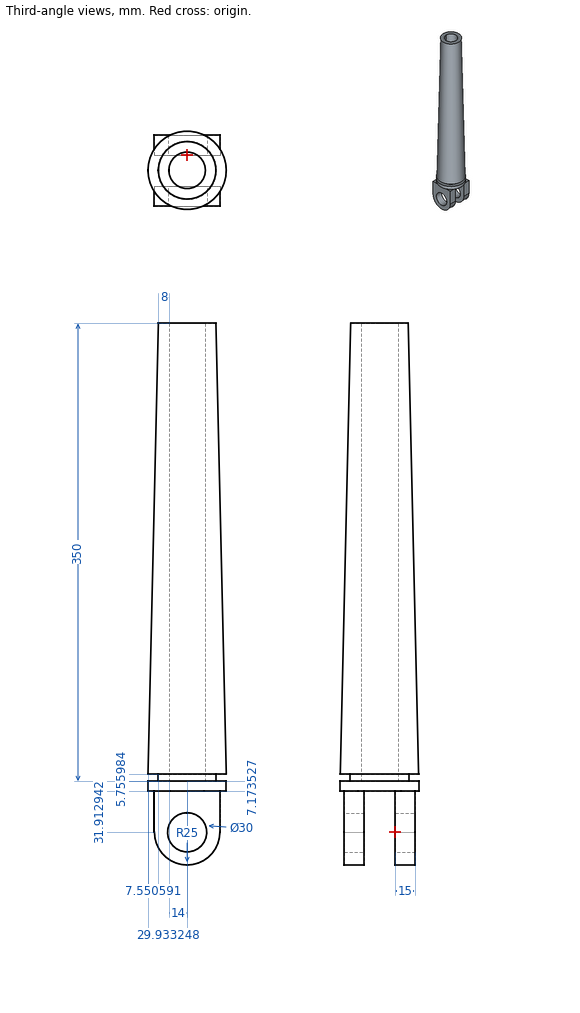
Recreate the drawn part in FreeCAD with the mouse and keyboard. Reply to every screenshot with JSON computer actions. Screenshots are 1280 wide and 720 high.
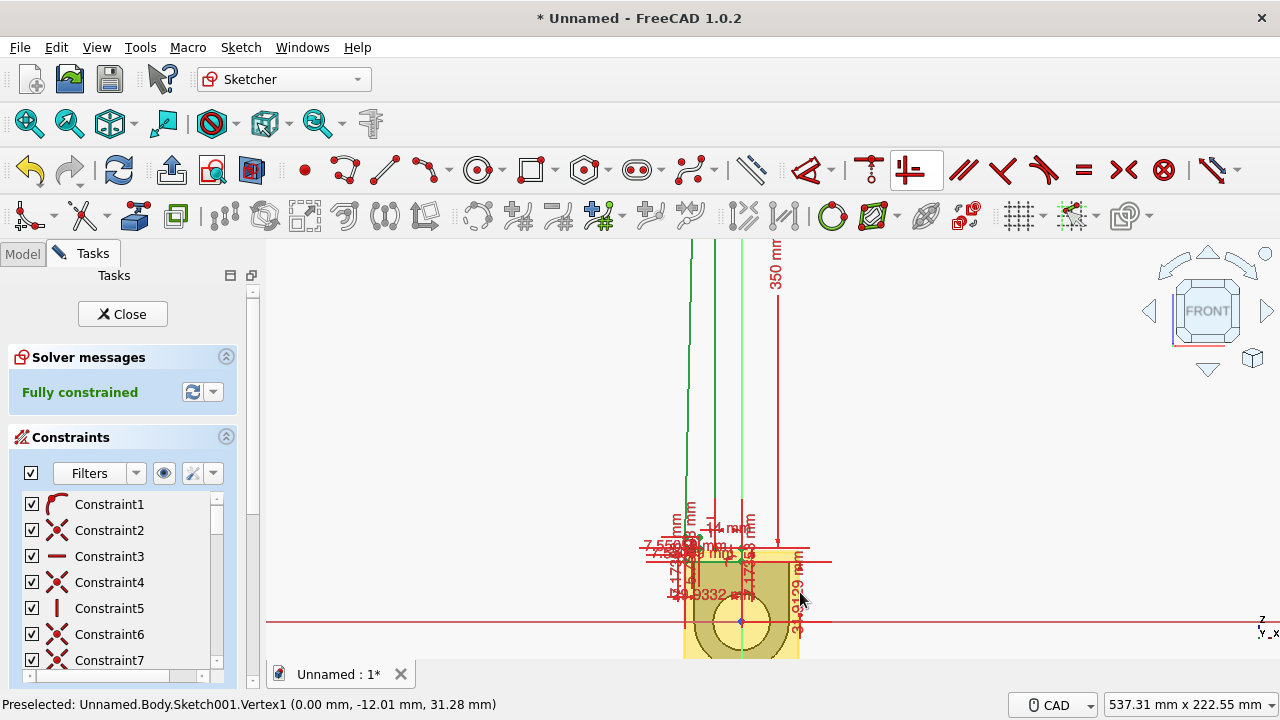
{"action": "left_click", "coordinate": [123, 314]}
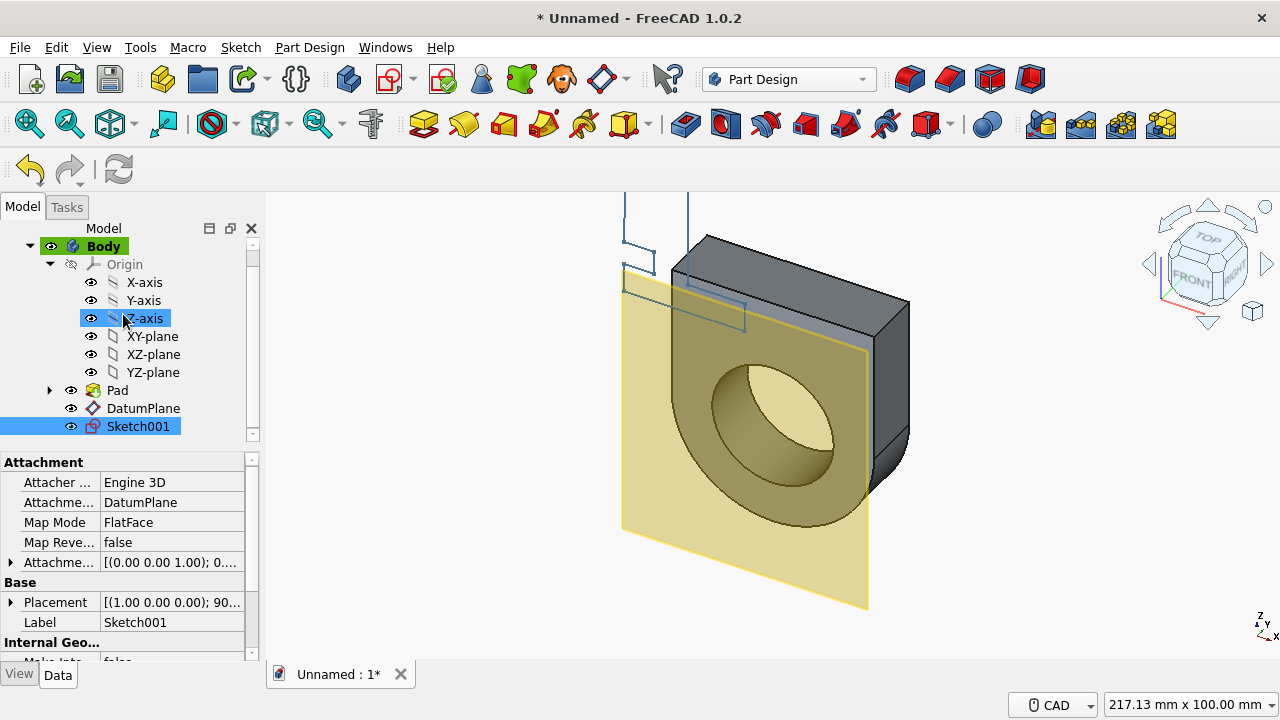
{"action": "left_click", "coordinate": [464, 124]}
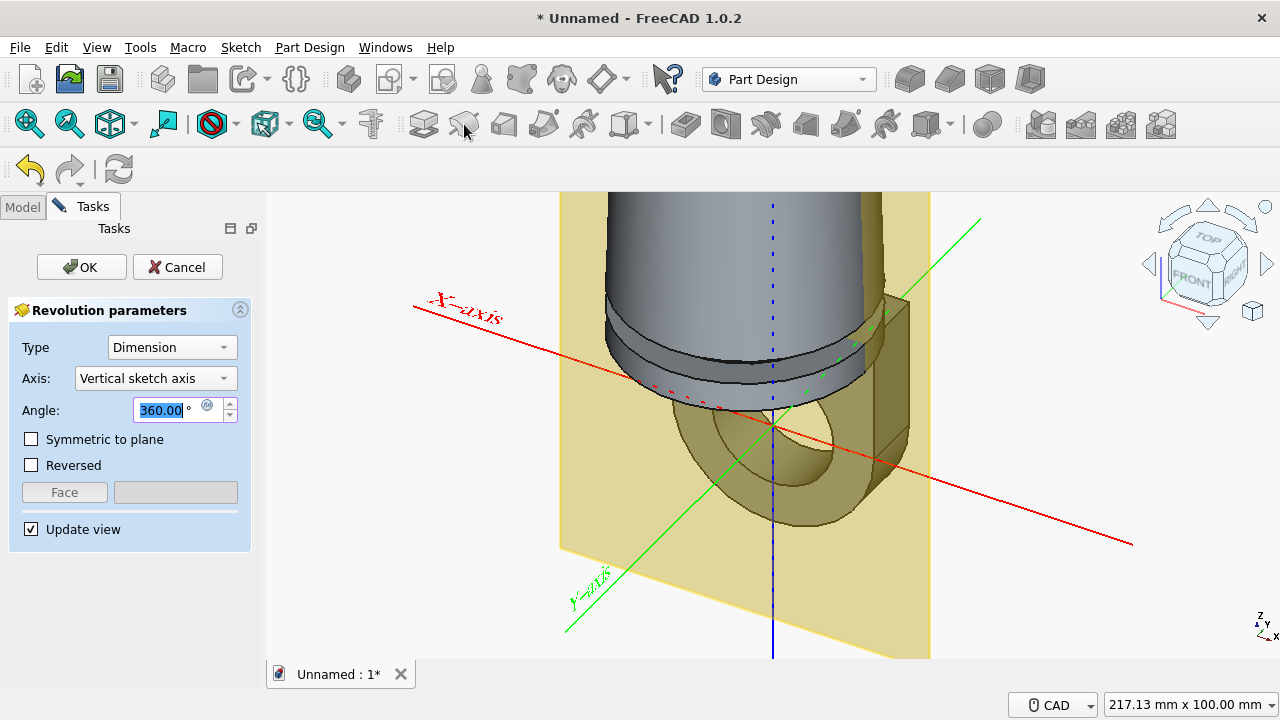
{"action": "left_click", "coordinate": [82, 267]}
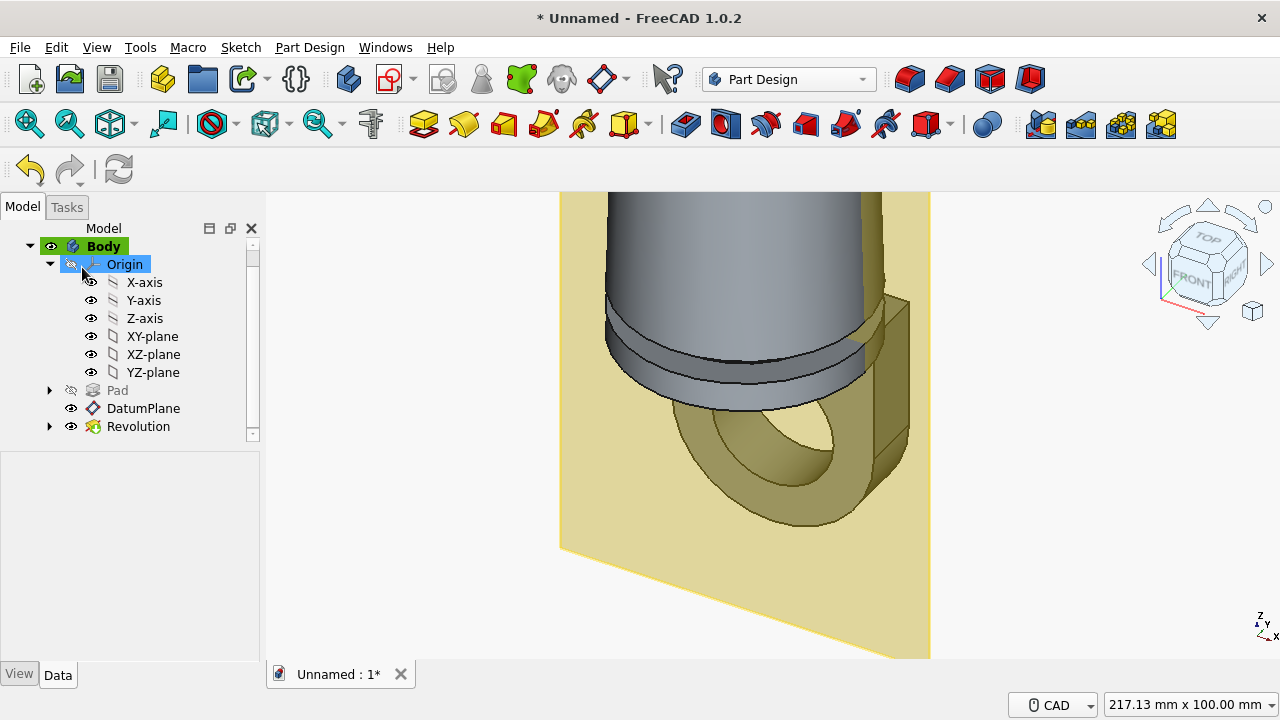
{"action": "left_click", "coordinate": [116, 408]}
{"action": "key", "text": "space"}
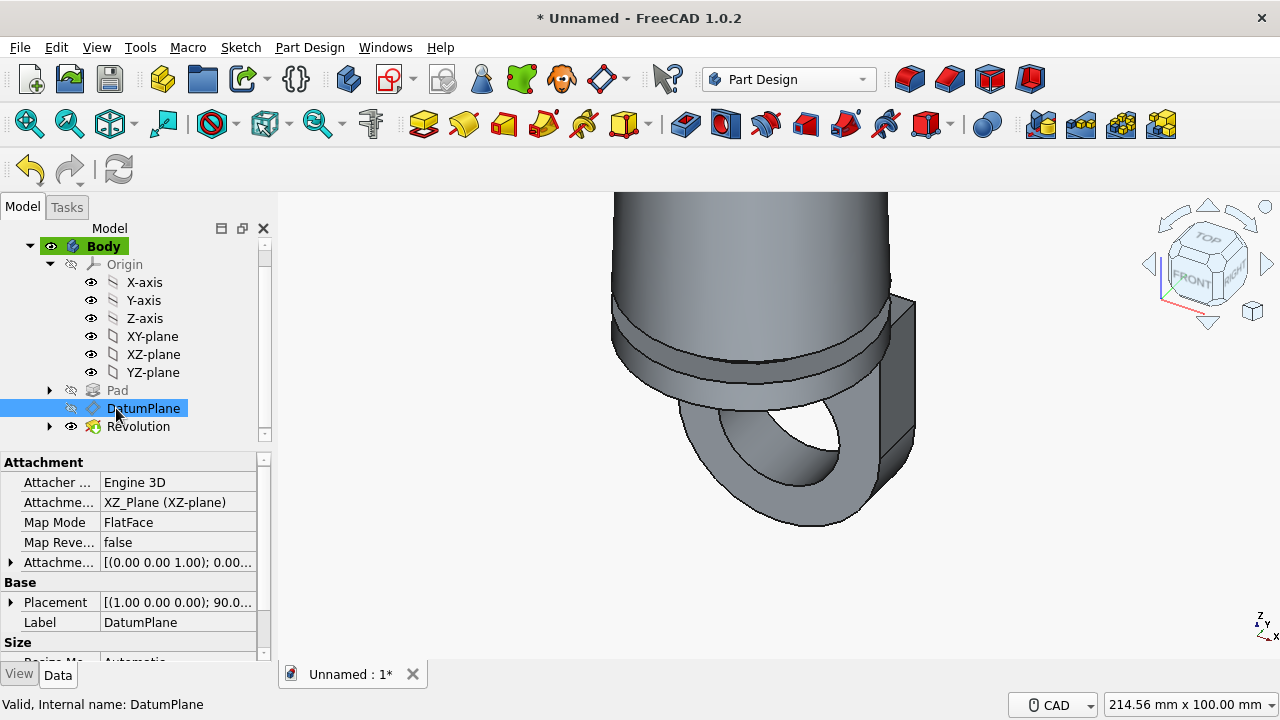
{"action": "left_click", "coordinate": [30, 124]}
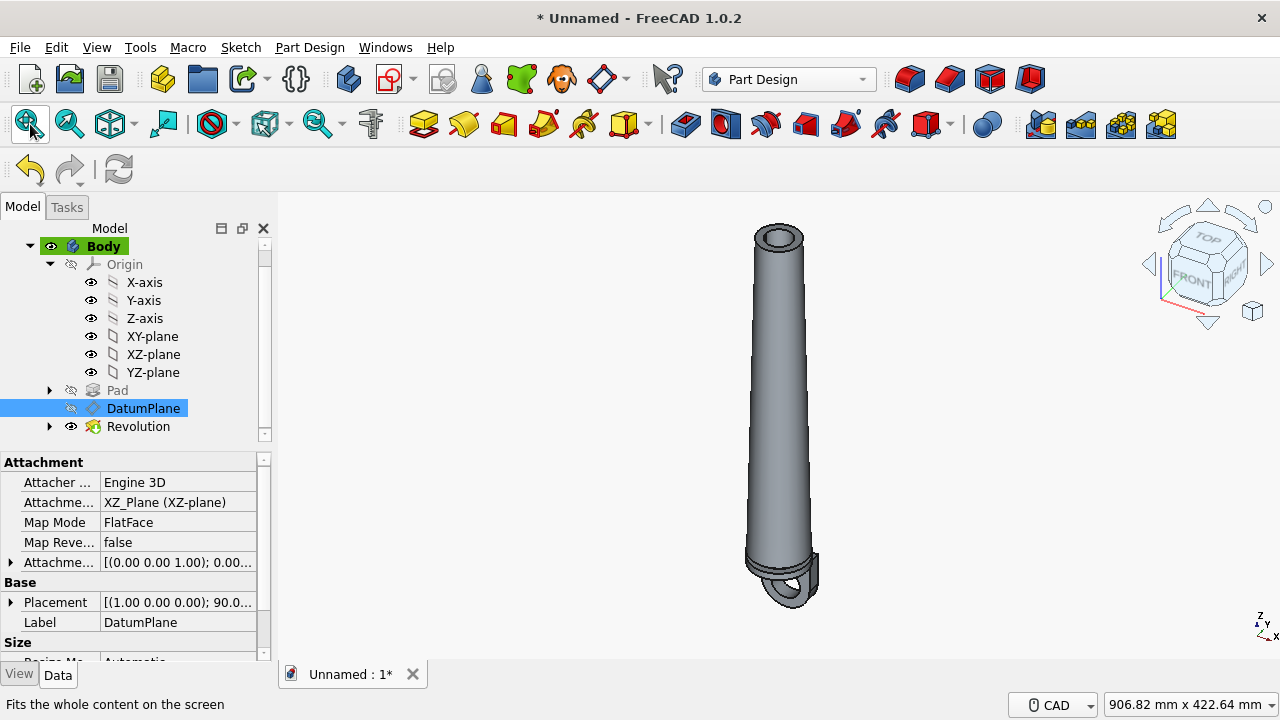
{"action": "left_click", "coordinate": [136, 354]}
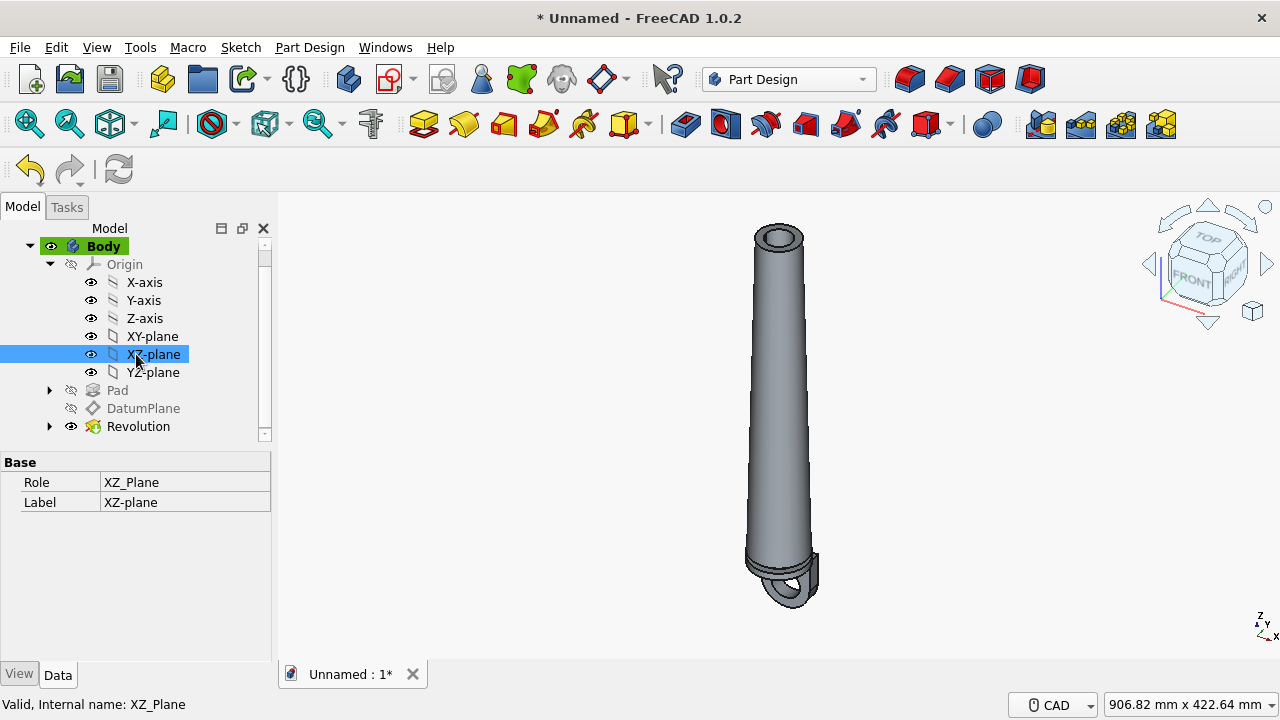
{"action": "left_click", "coordinate": [602, 80]}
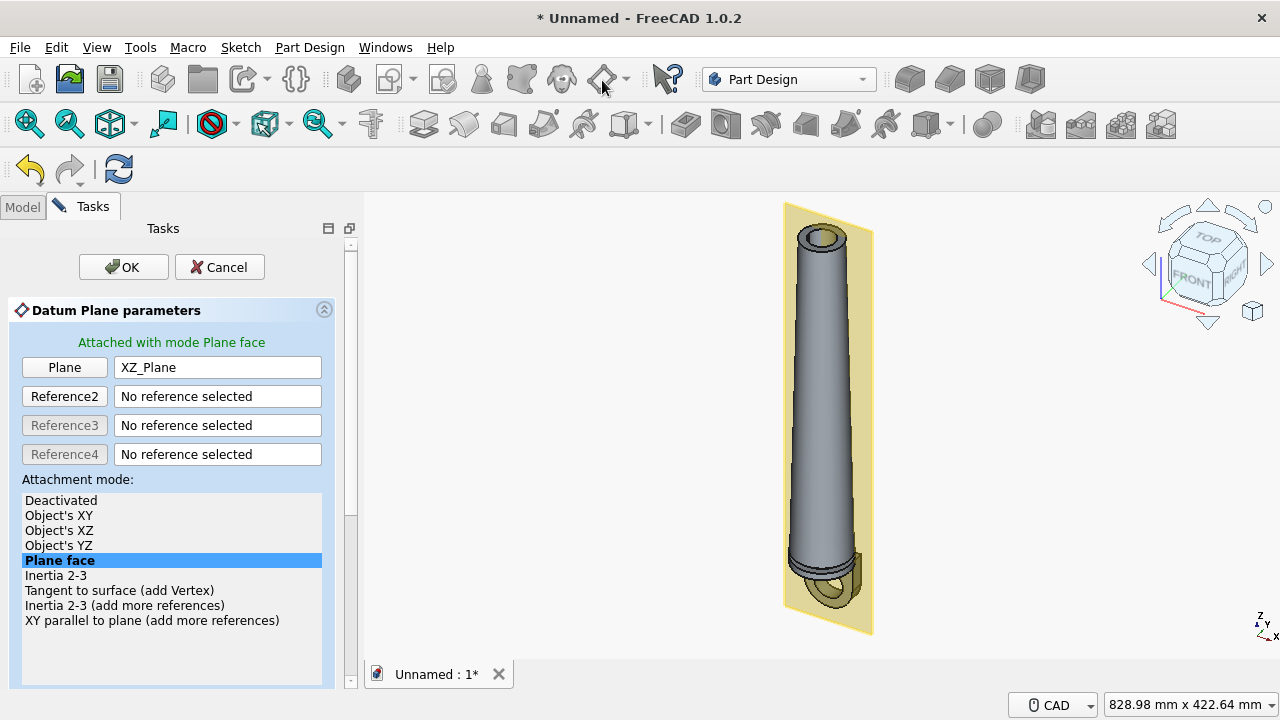
{"action": "scroll", "coordinate": [351, 463], "scroll_direction": "down", "scroll_amount": 3}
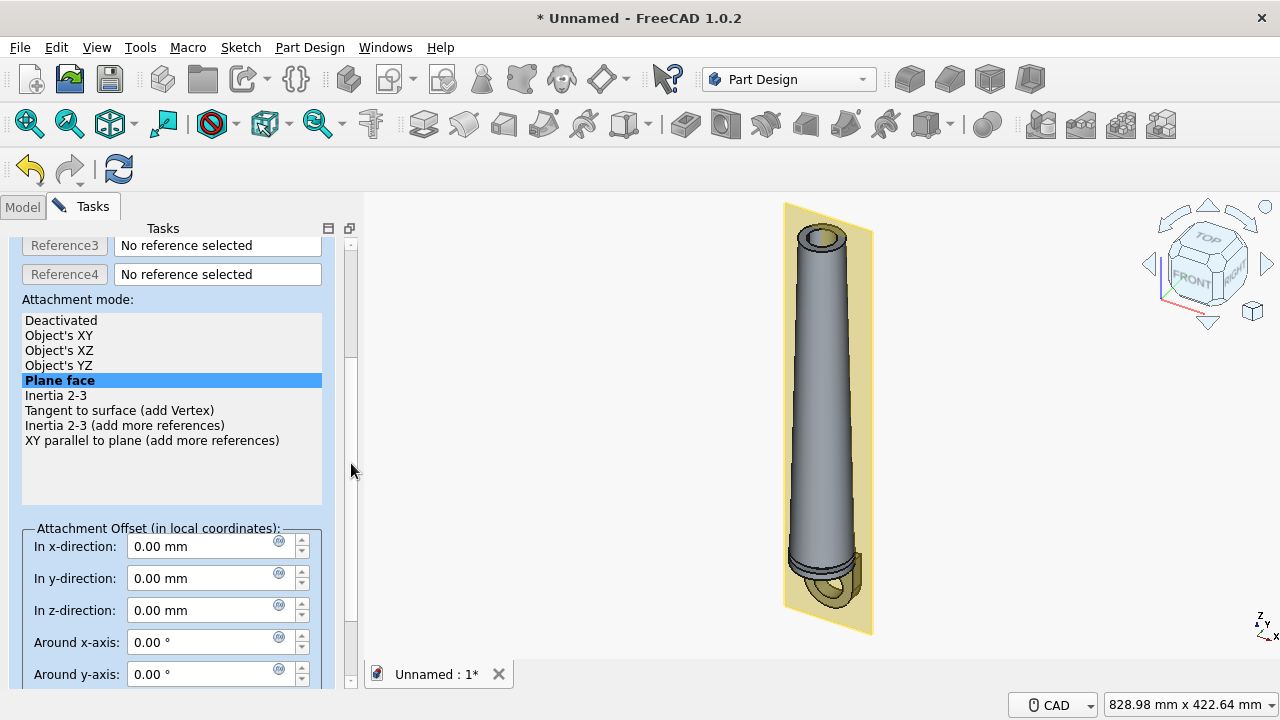
{"action": "triple_click", "coordinate": [210, 610]}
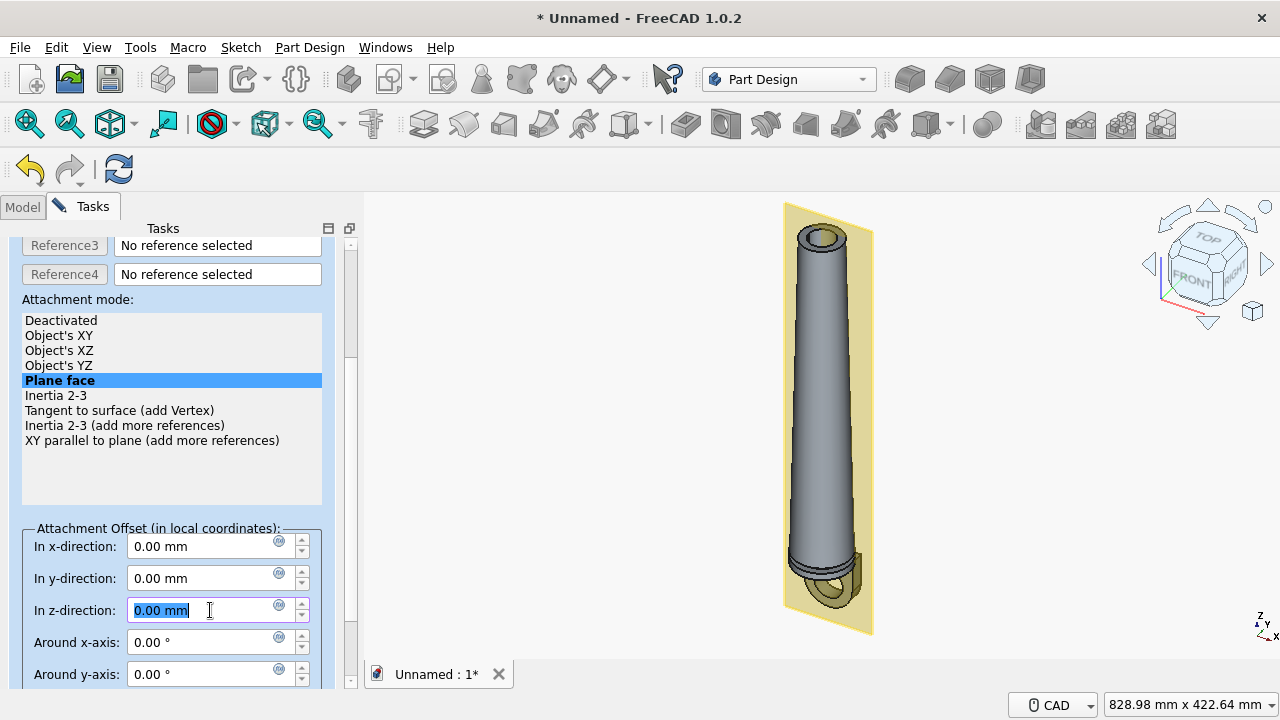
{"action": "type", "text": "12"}
{"action": "key", "text": "Tab"}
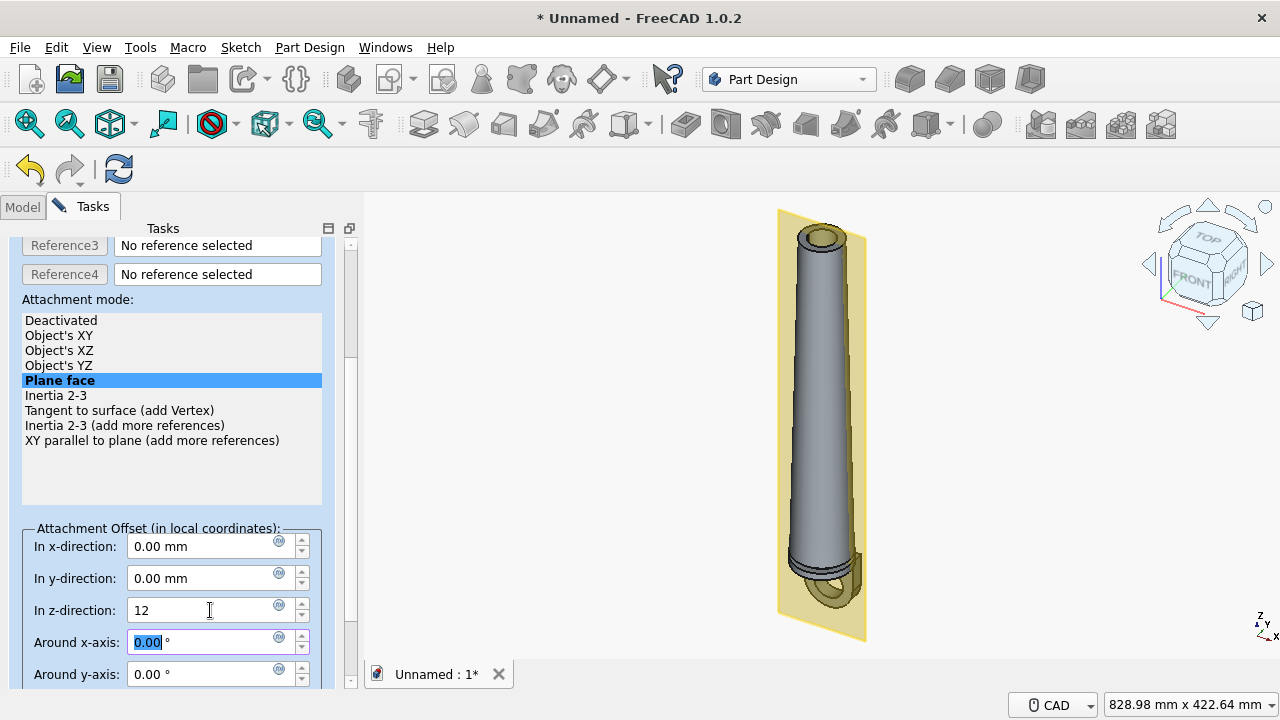
{"action": "scroll", "coordinate": [351, 463], "scroll_direction": "up", "scroll_amount": 4}